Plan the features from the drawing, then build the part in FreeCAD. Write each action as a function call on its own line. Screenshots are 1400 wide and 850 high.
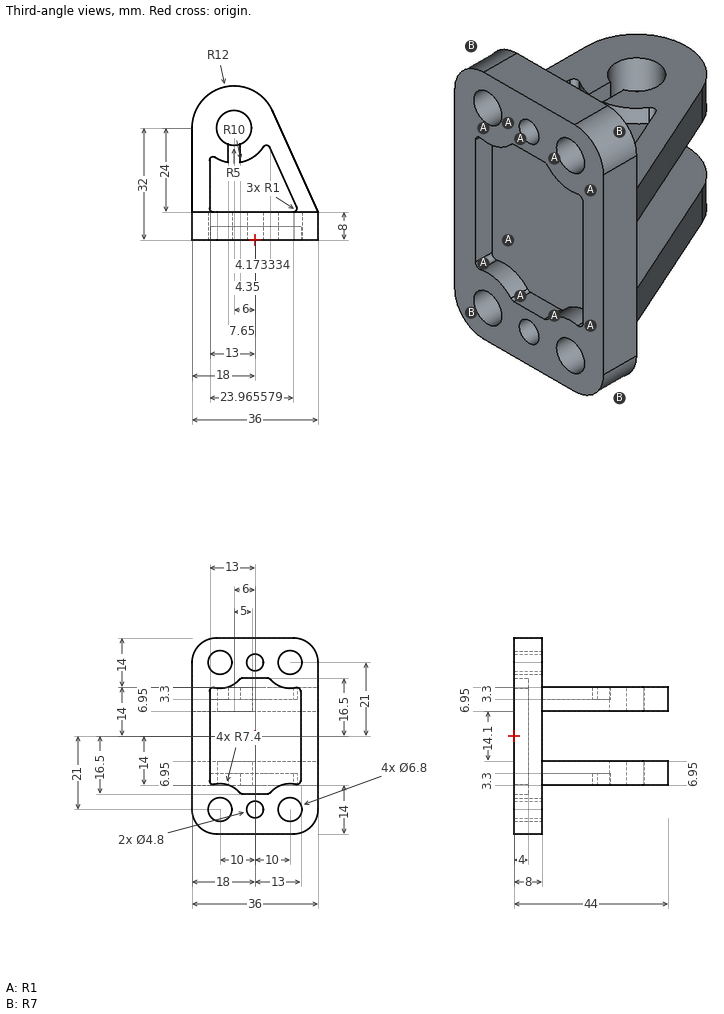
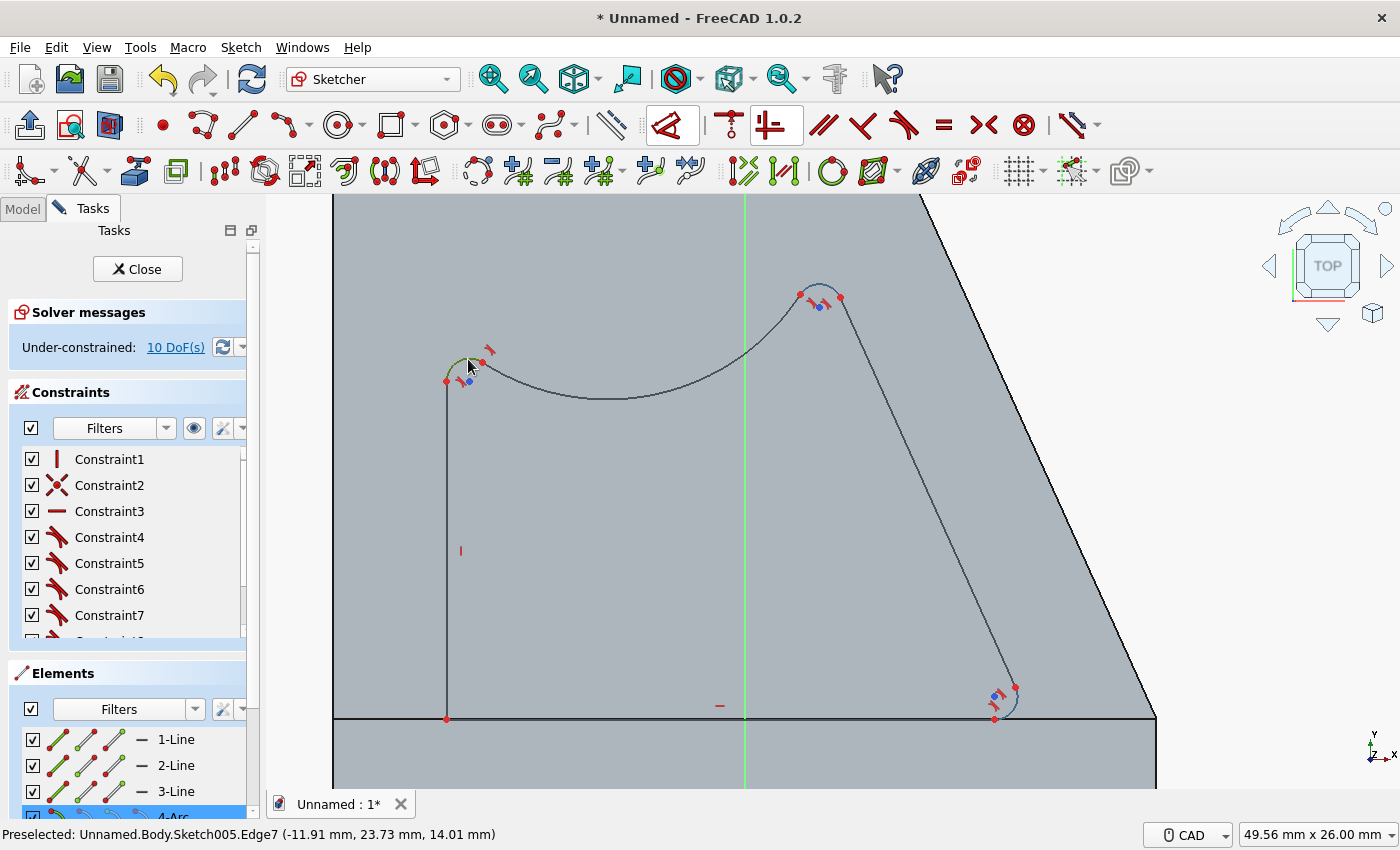
click(944, 126)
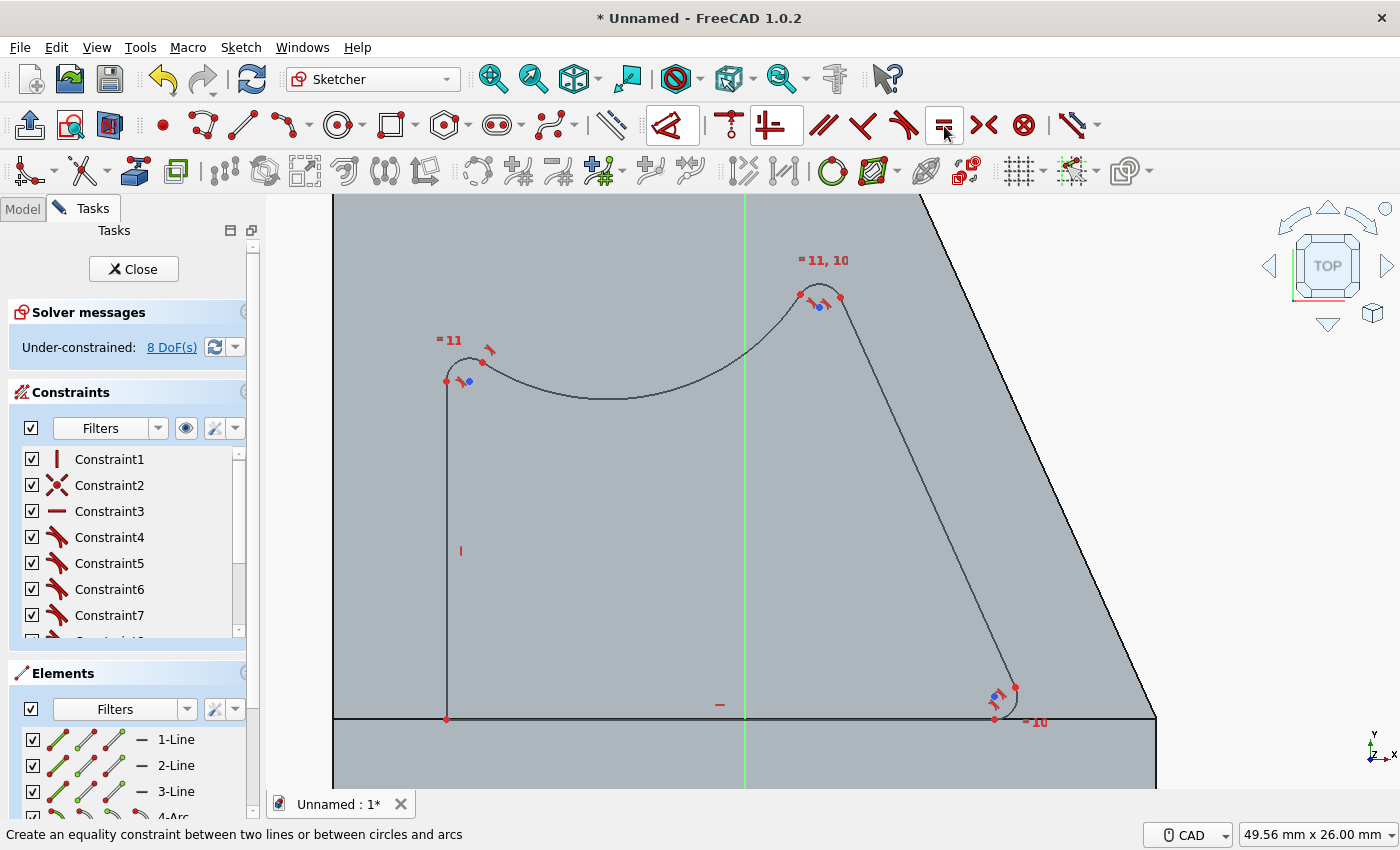
scroll(1007, 716, up, 3)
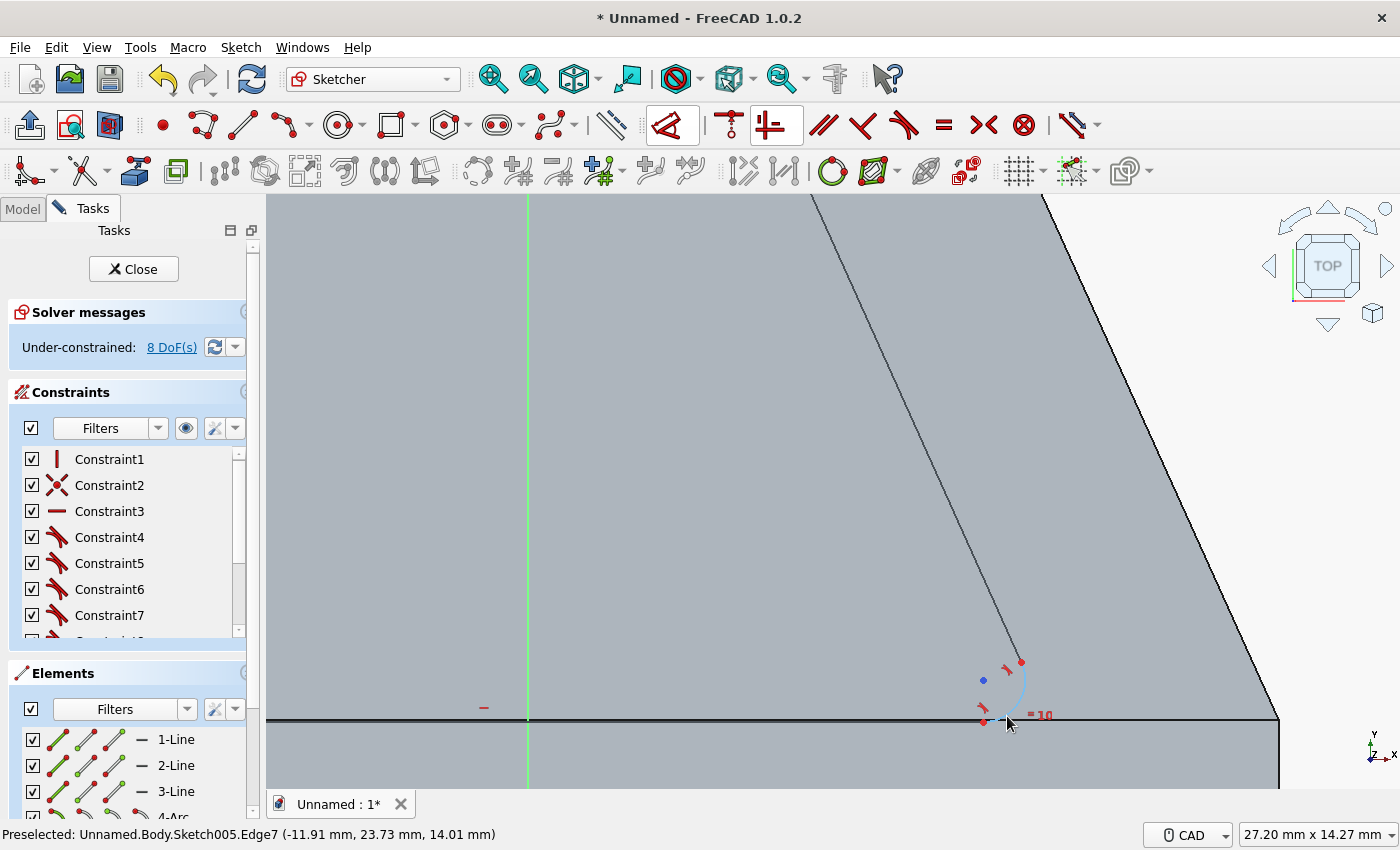
click(1007, 715)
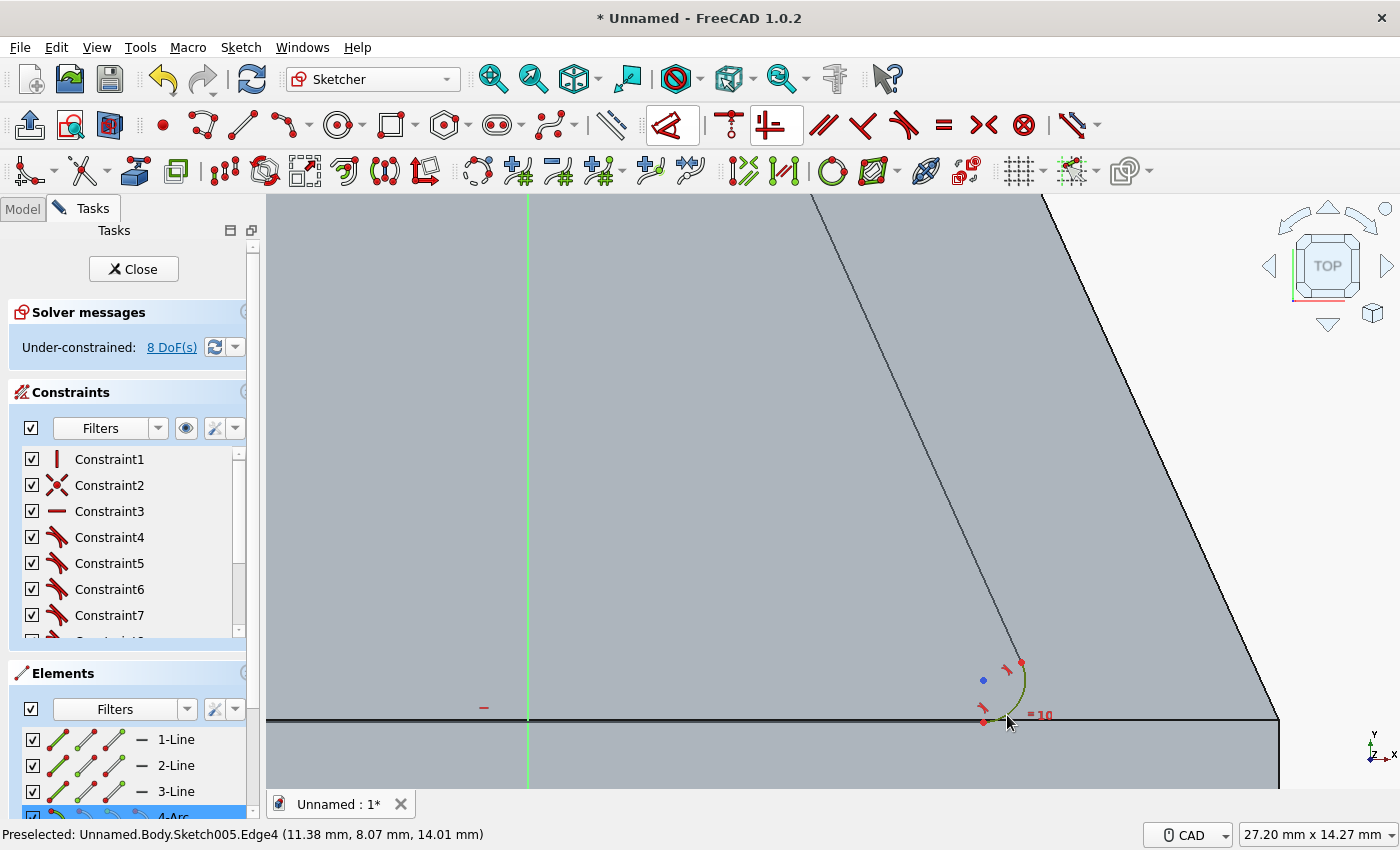
key(k)
key(r)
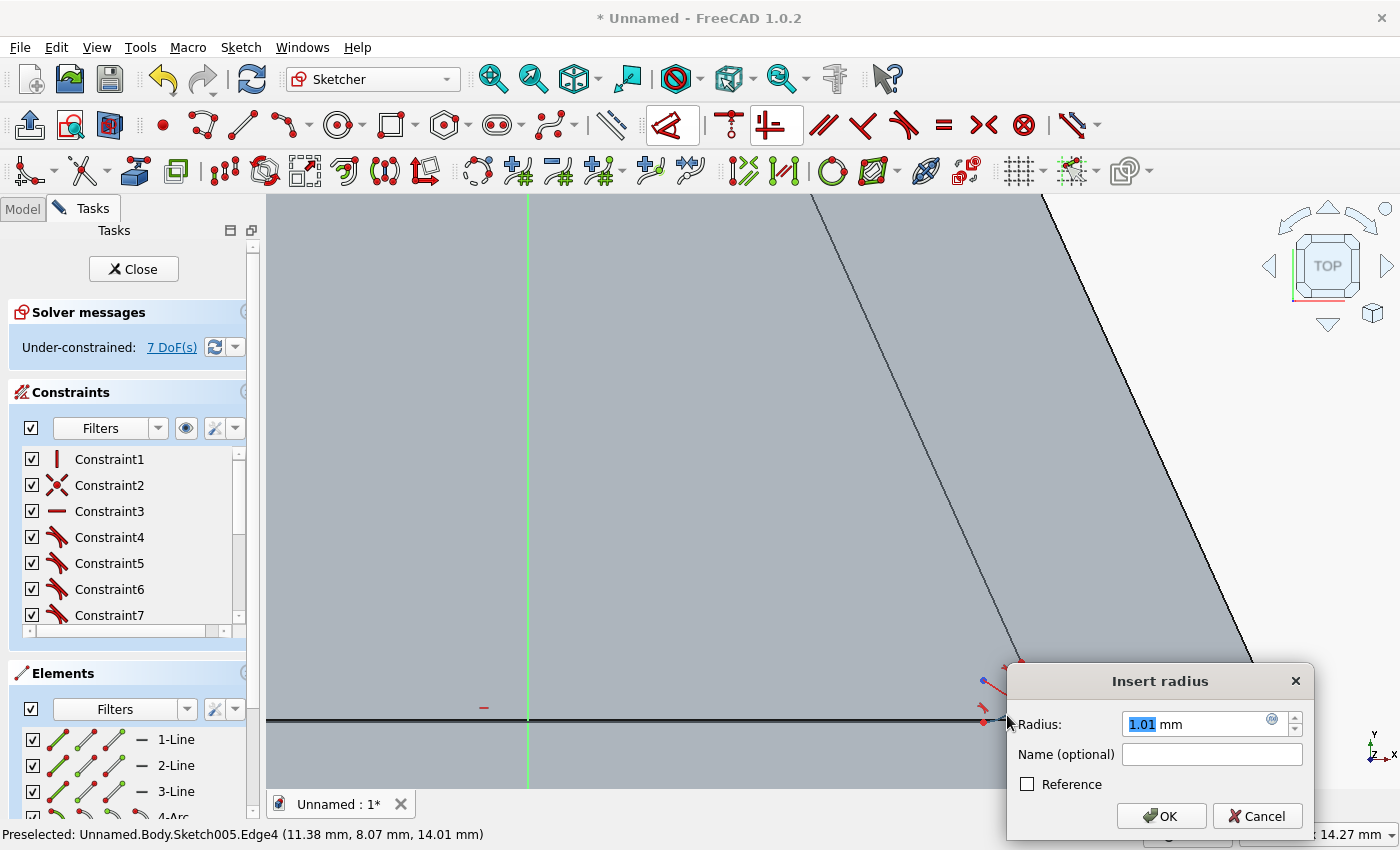
text(1)
key(Return)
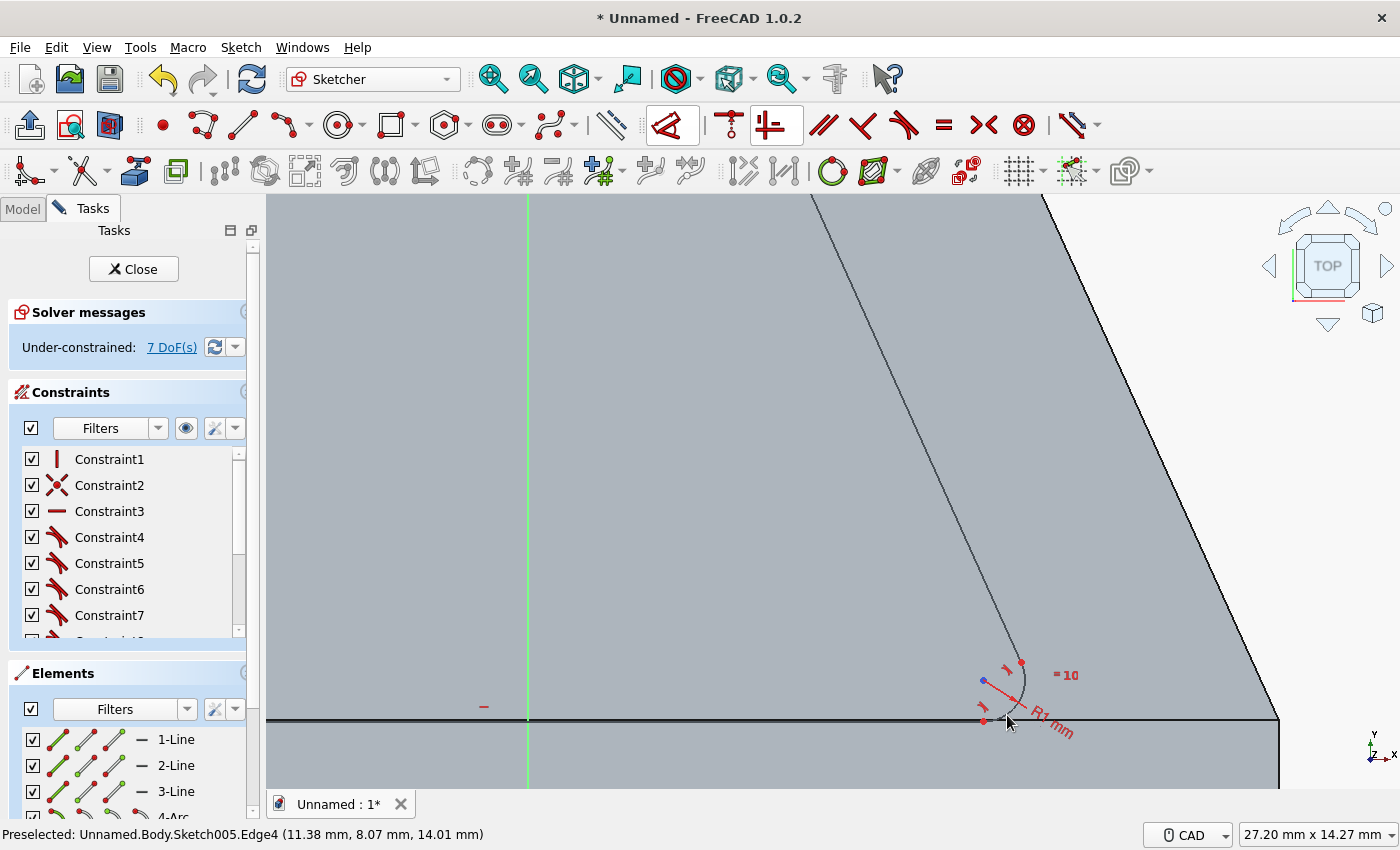
scroll(916, 493, down, 5)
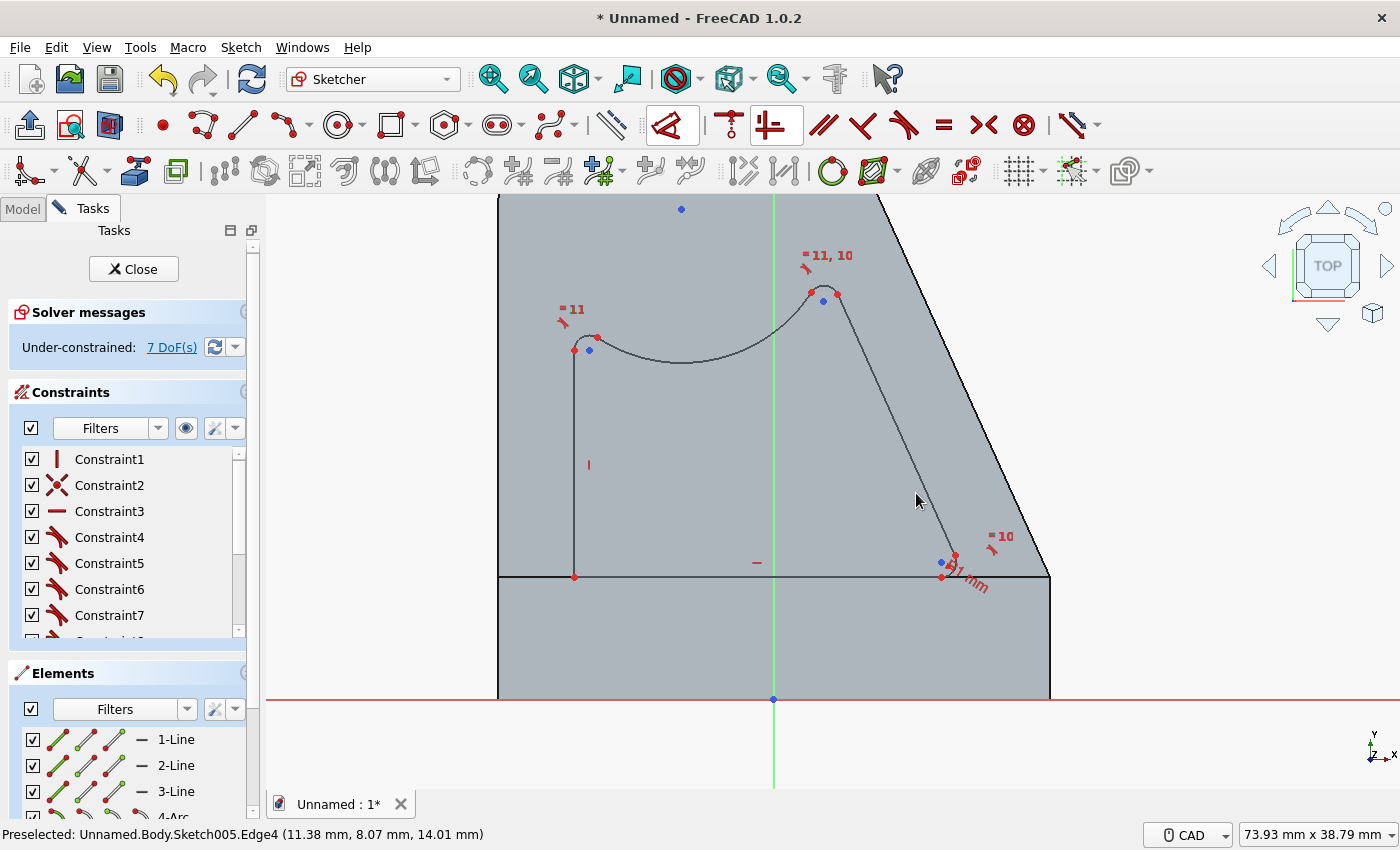
click(666, 362)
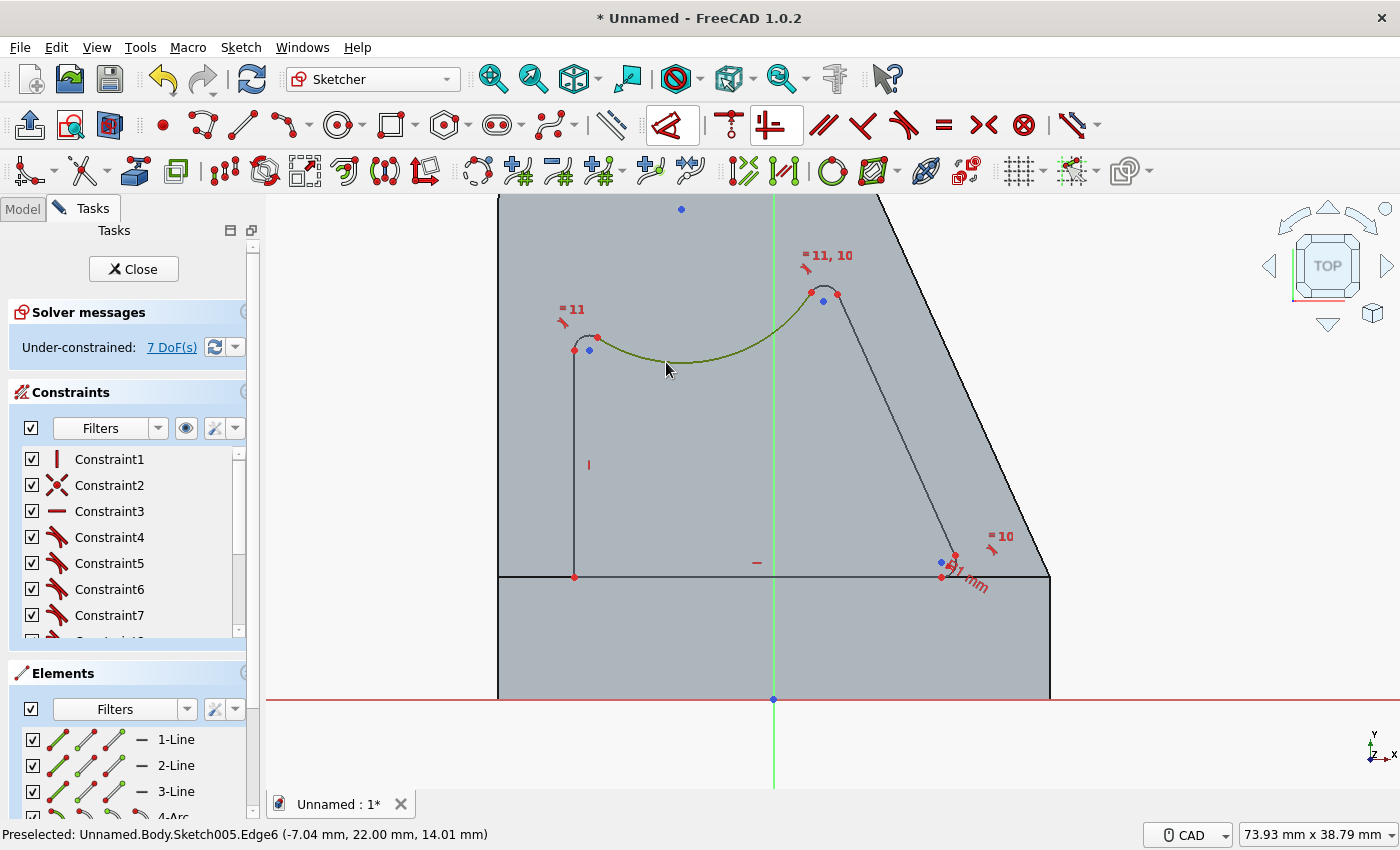
key(k)
key(r)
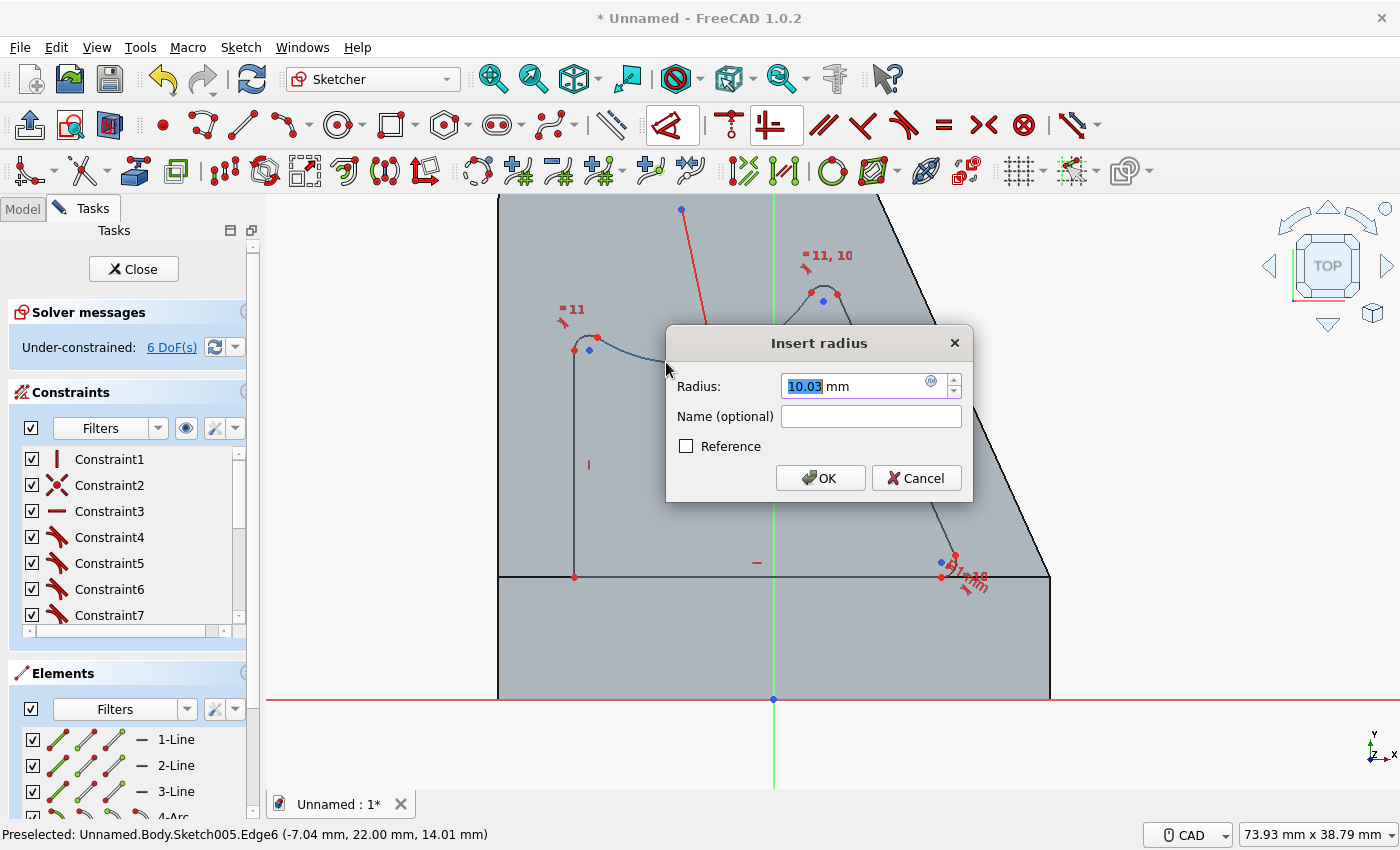
text(10)
key(Return)